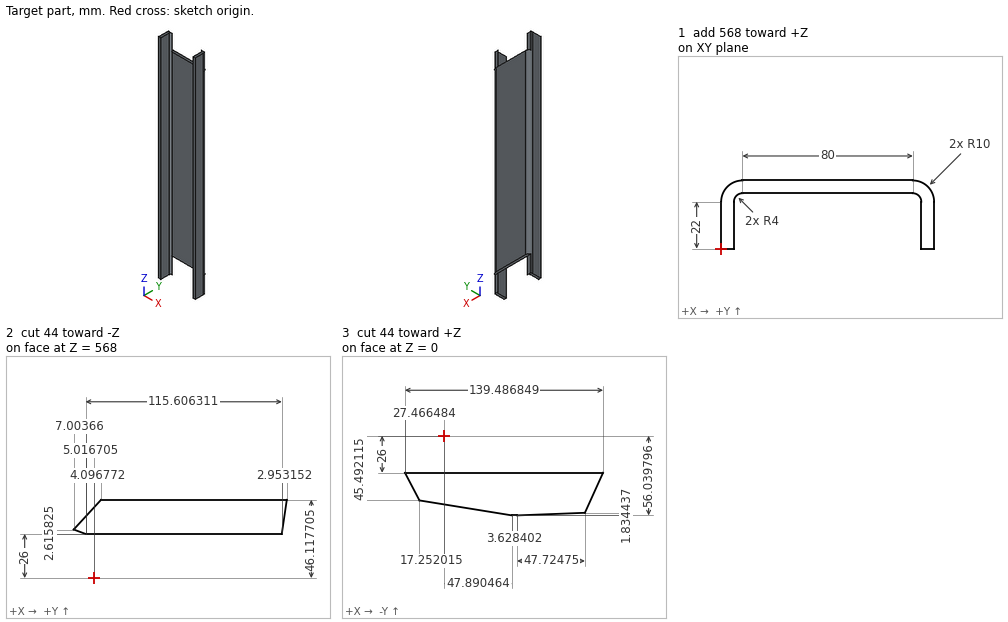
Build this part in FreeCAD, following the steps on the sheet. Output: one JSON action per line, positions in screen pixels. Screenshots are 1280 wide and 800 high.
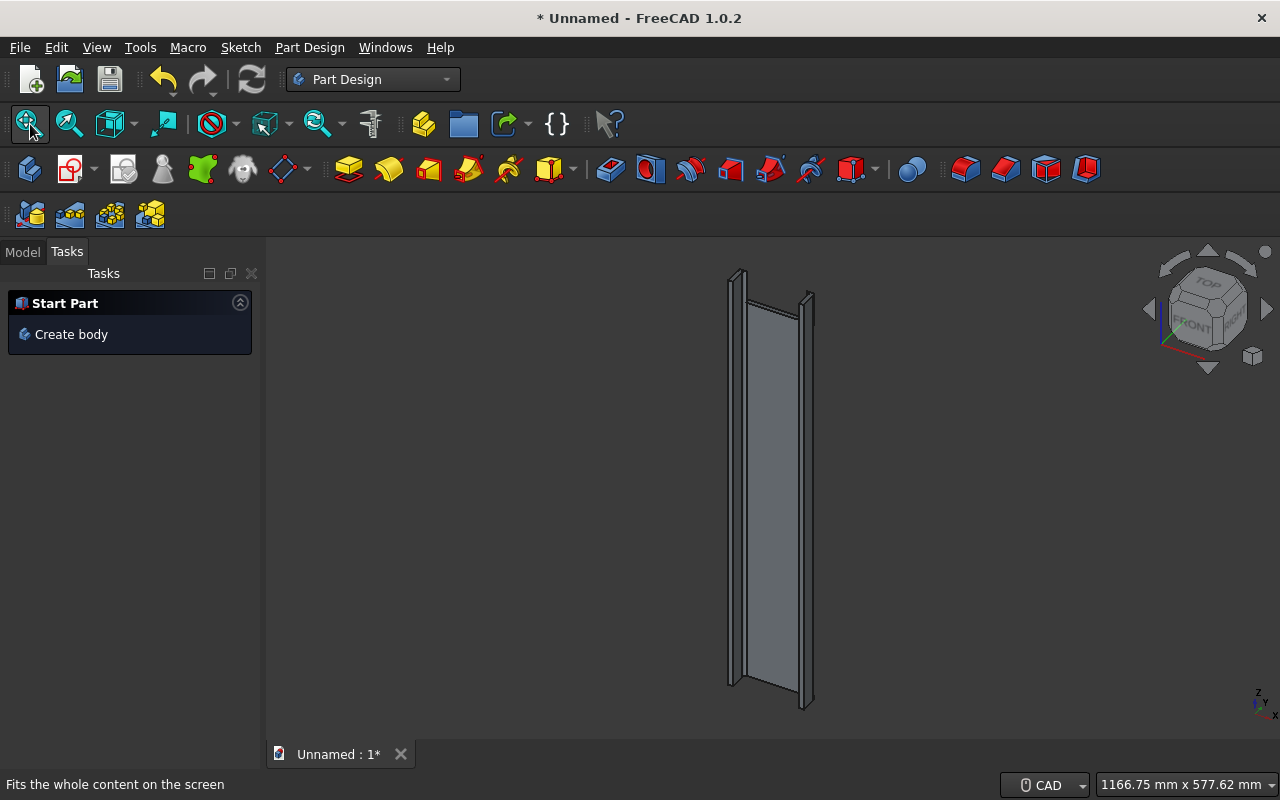
{"action": "key", "text": "5"}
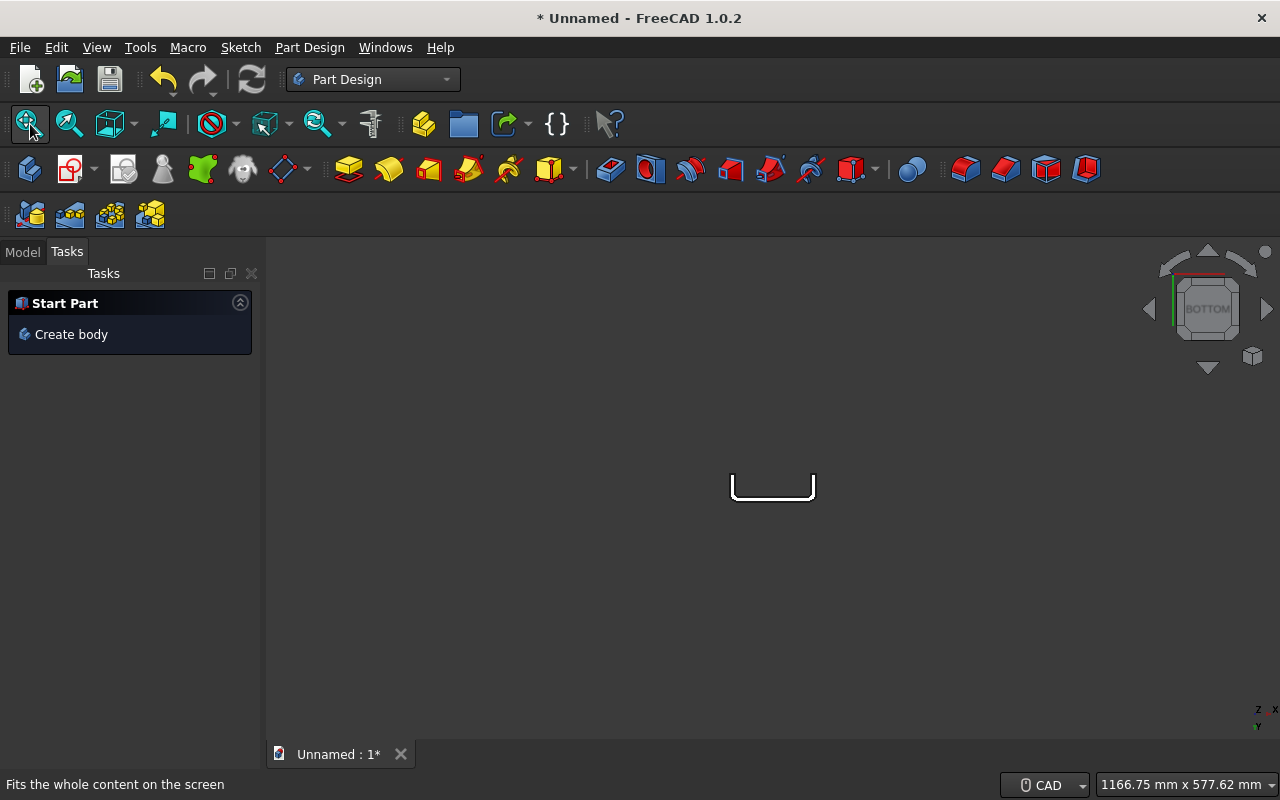
{"action": "left_click", "coordinate": [30, 124]}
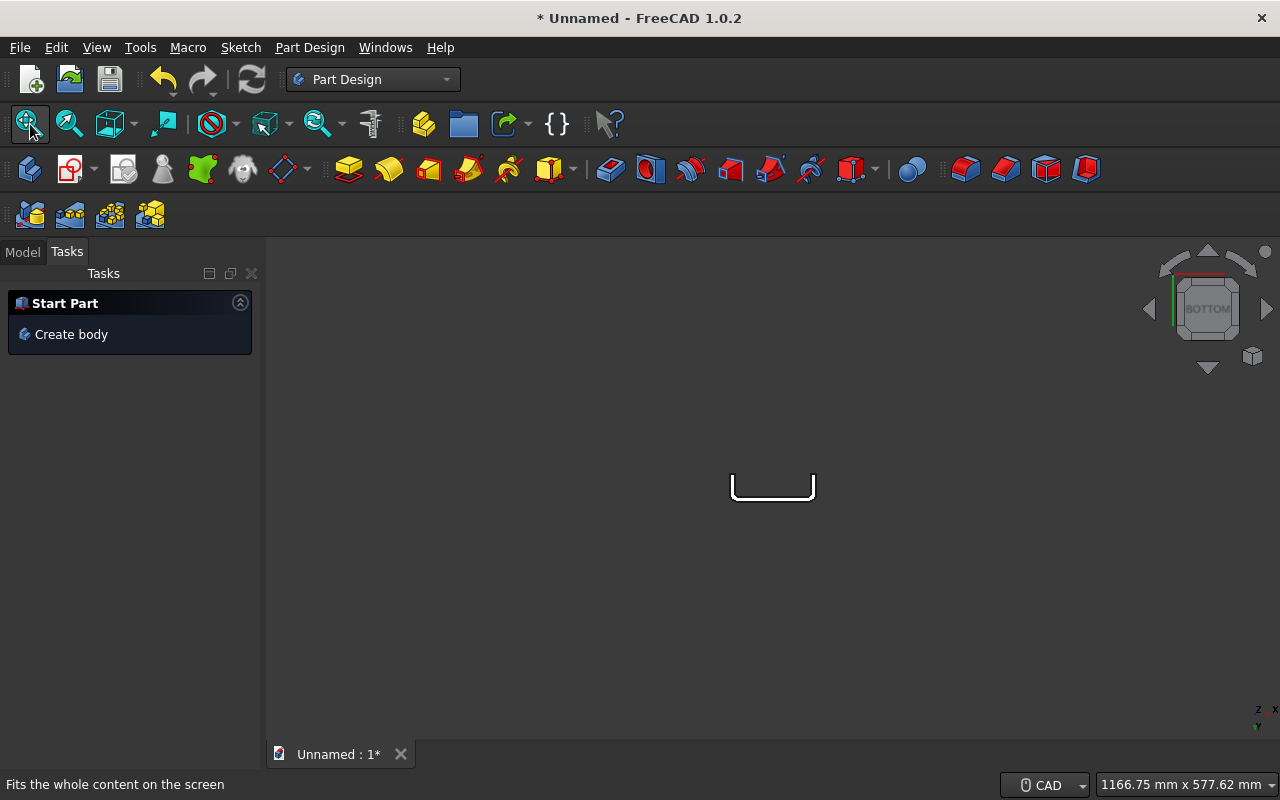
{"action": "scroll", "coordinate": [798, 499], "scroll_direction": "up", "scroll_amount": 9}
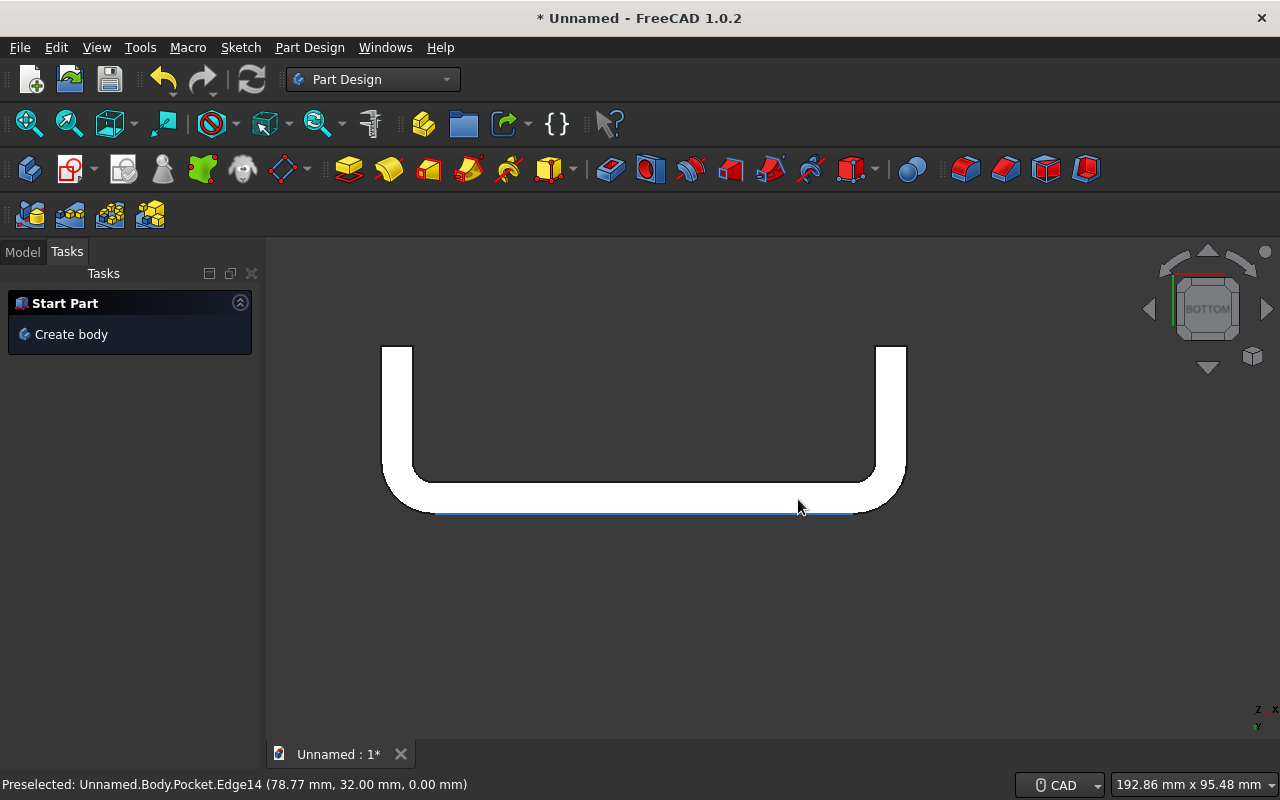
{"action": "left_click", "coordinate": [794, 501]}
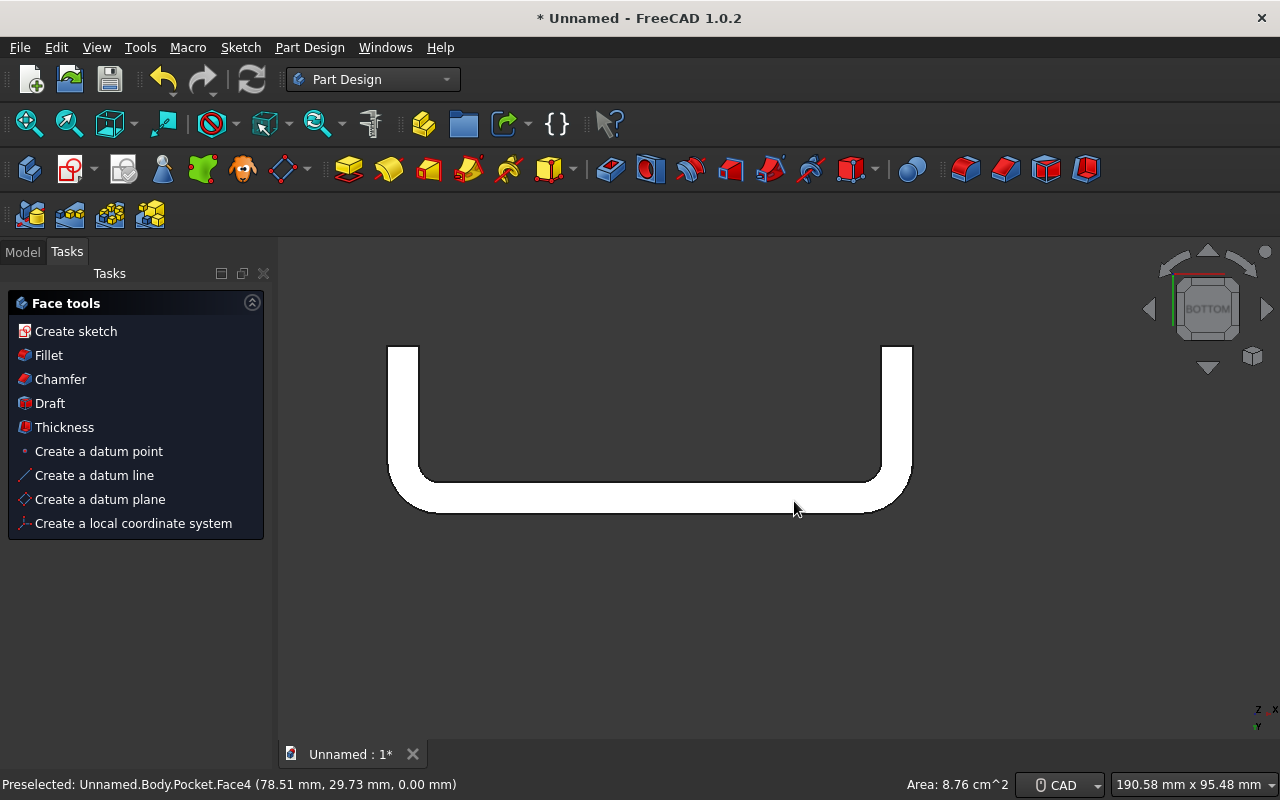
{"action": "left_click", "coordinate": [70, 170]}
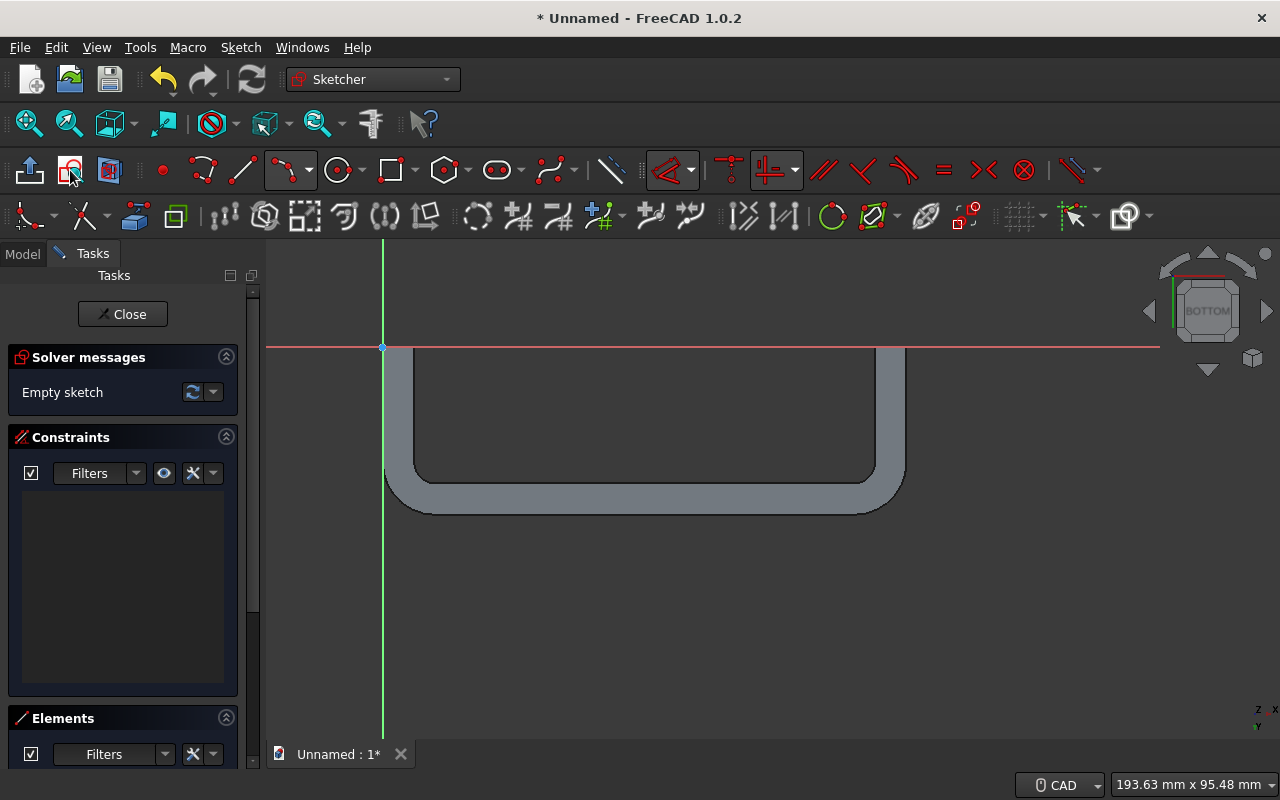
{"action": "scroll", "coordinate": [1115, 466], "scroll_direction": "down", "scroll_amount": 1}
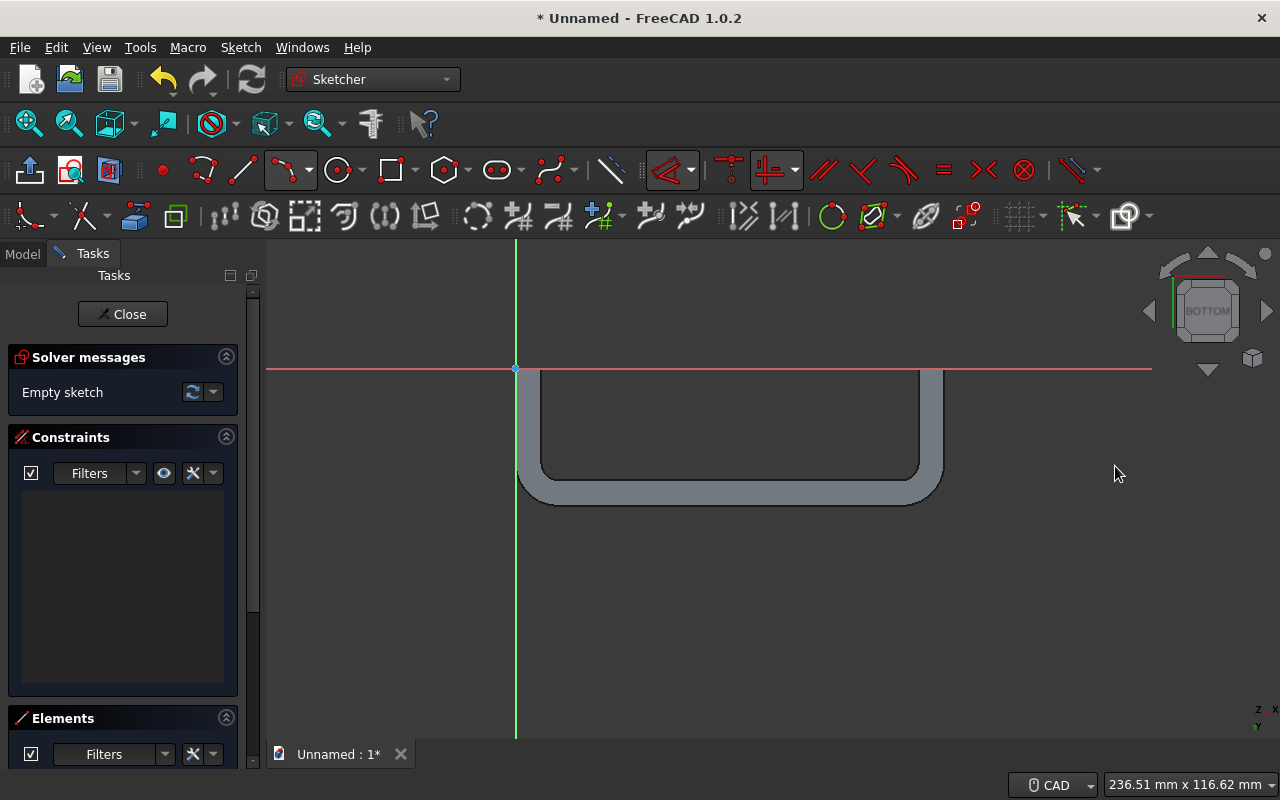
{"action": "left_click", "coordinate": [204, 170]}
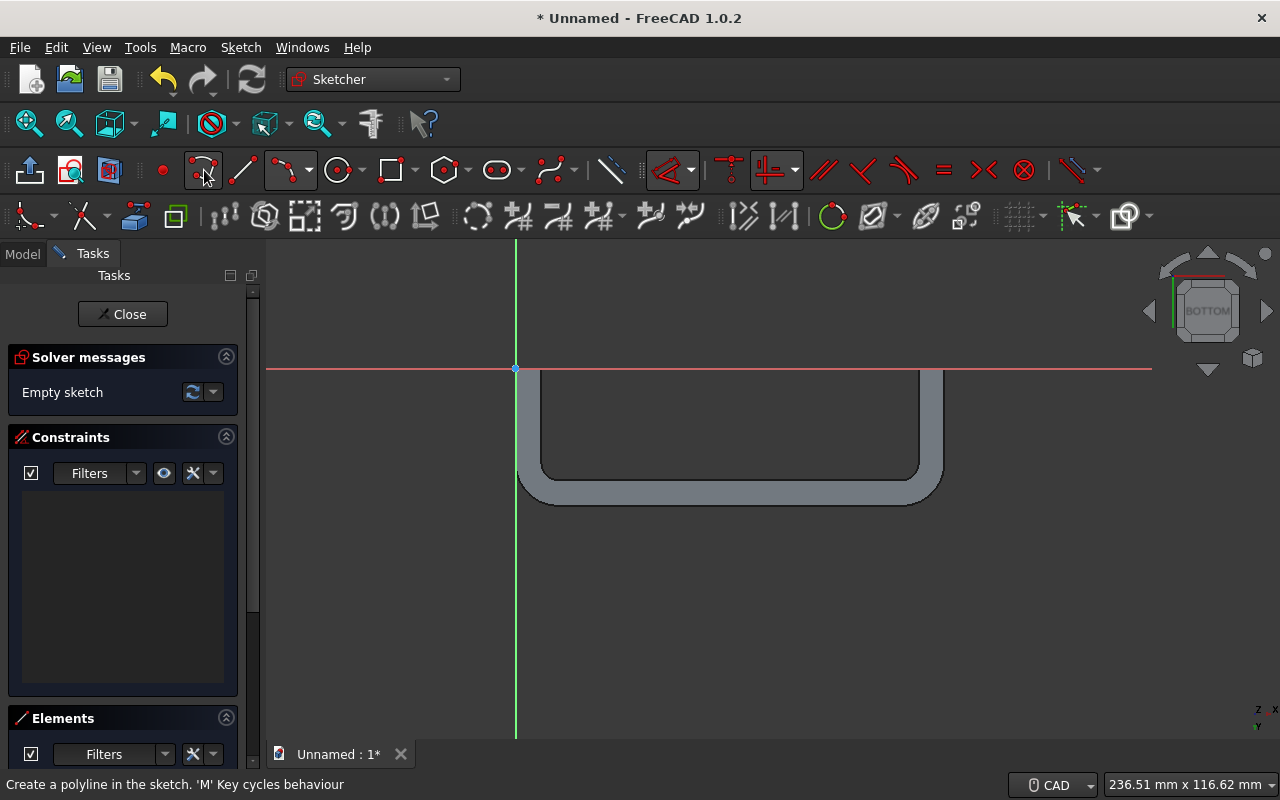
{"action": "left_click", "coordinate": [398, 480]}
{"action": "left_click", "coordinate": [442, 564]}
{"action": "left_click", "coordinate": [721, 609]}
{"action": "left_click", "coordinate": [737, 609]}
{"action": "left_click", "coordinate": [941, 598]}
{"action": "left_click", "coordinate": [996, 480]}
{"action": "left_click", "coordinate": [398, 481]}
{"action": "key", "text": "Escape"}
{"action": "key", "text": "Escape"}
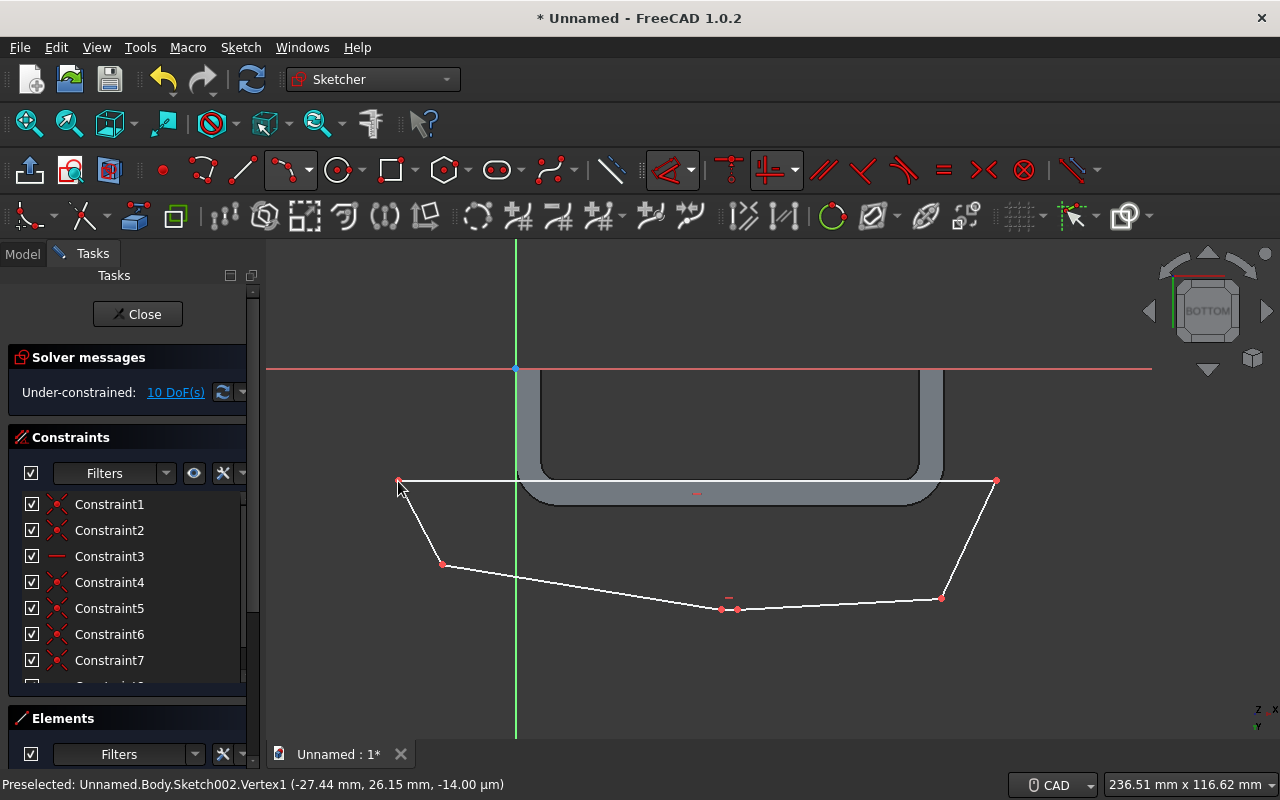
{"action": "left_click", "coordinate": [398, 481]}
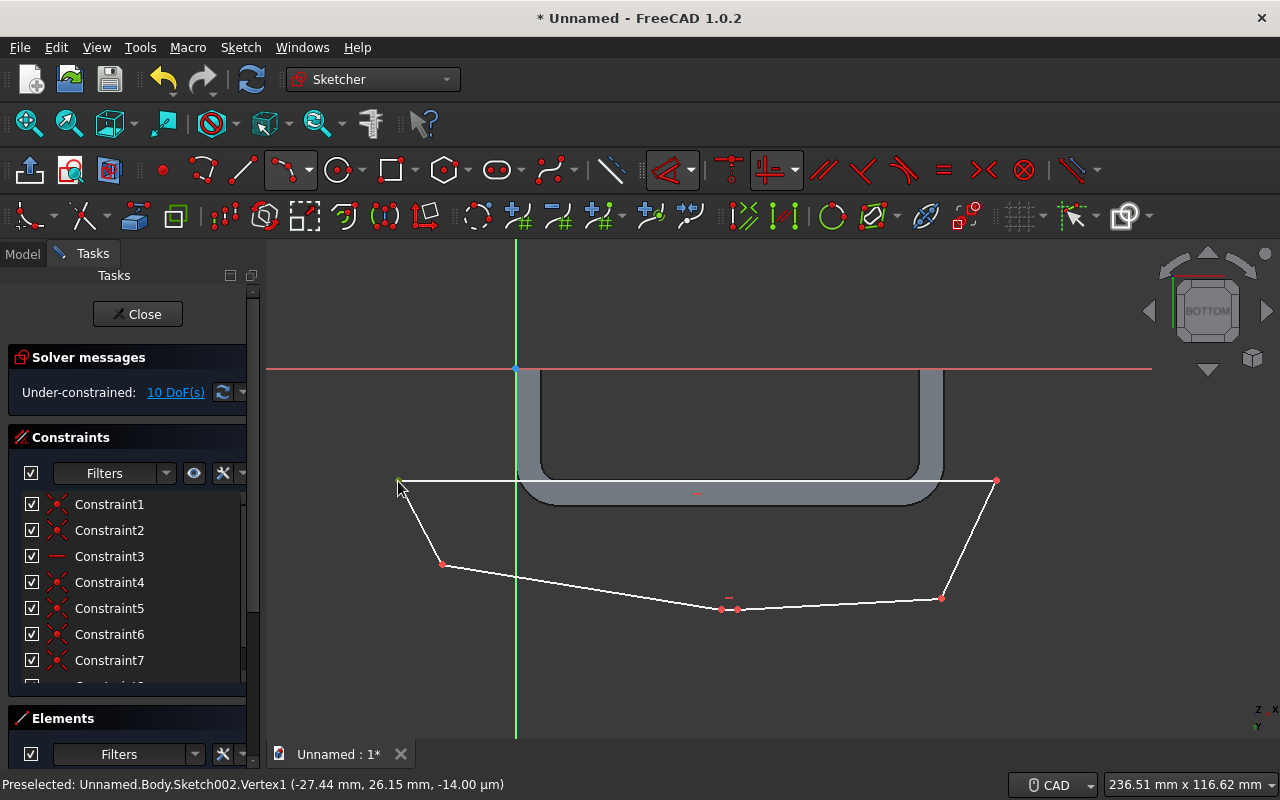
{"action": "key", "text": "i"}